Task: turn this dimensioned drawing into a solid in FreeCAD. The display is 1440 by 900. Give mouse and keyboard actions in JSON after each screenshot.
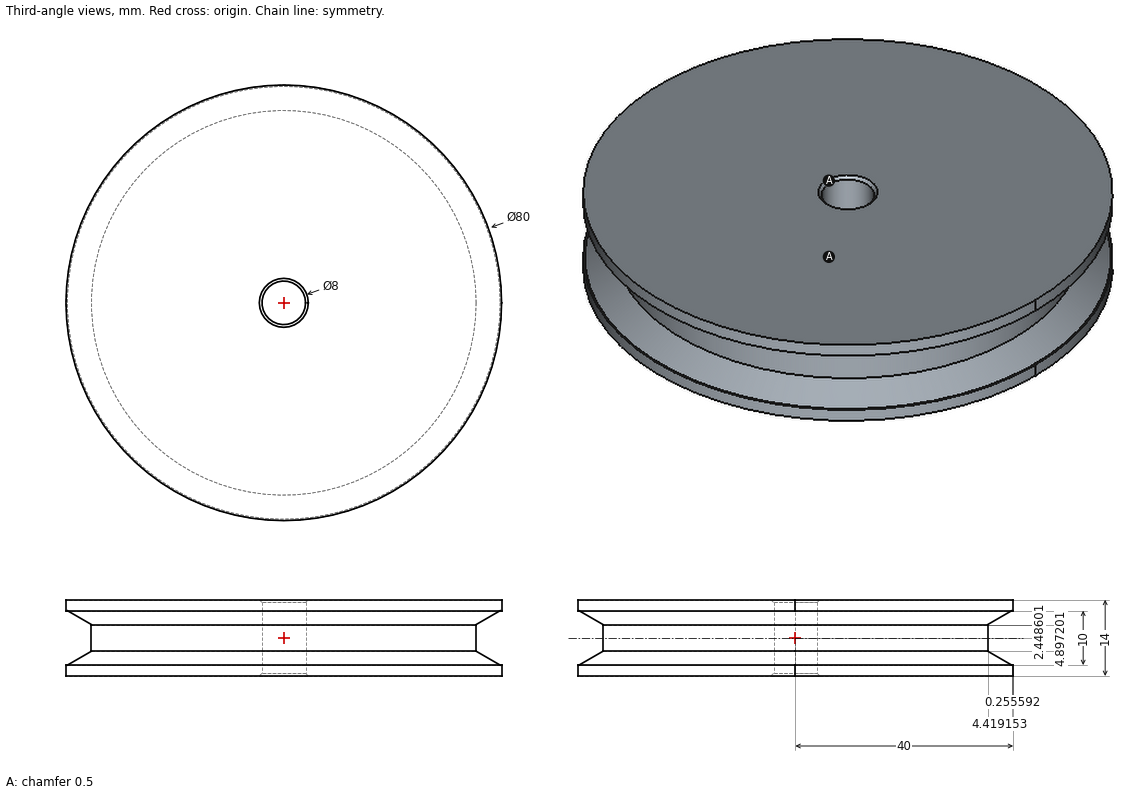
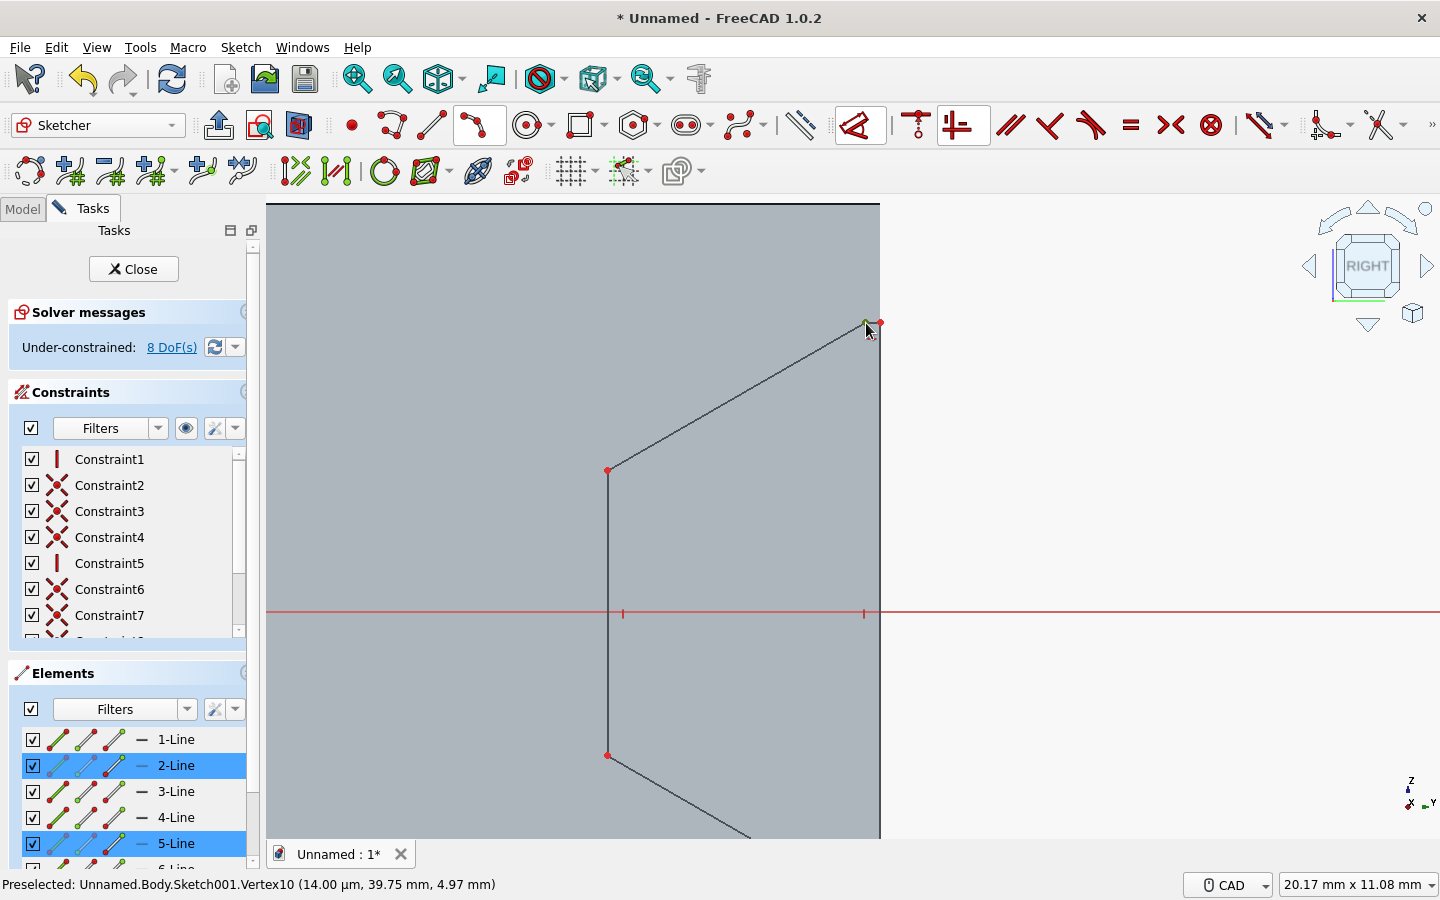
{"action": "left_click", "coordinate": [364, 612]}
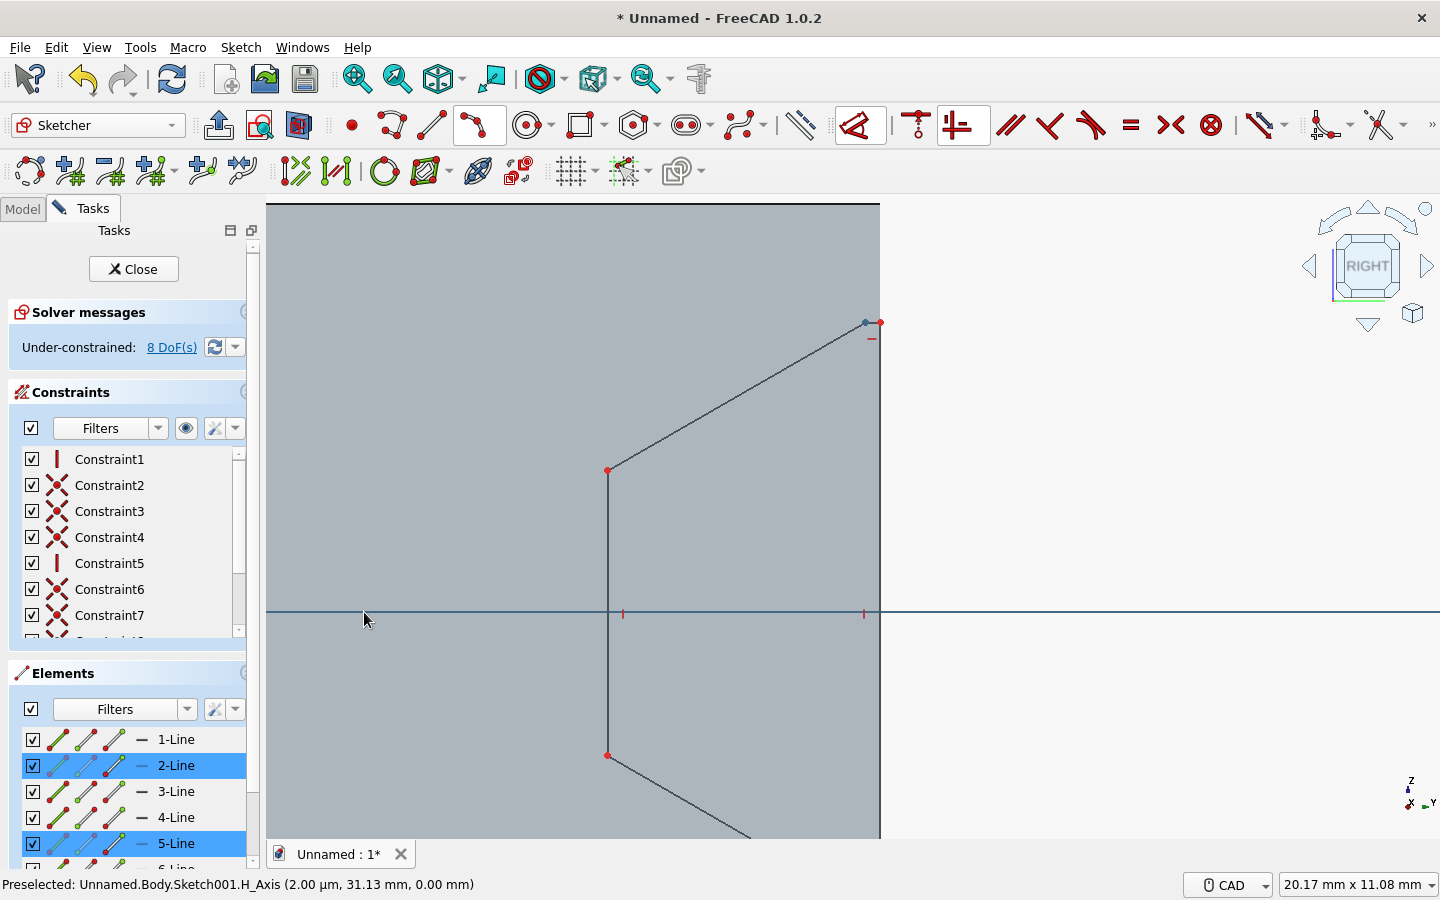
{"action": "left_click", "coordinate": [1172, 126]}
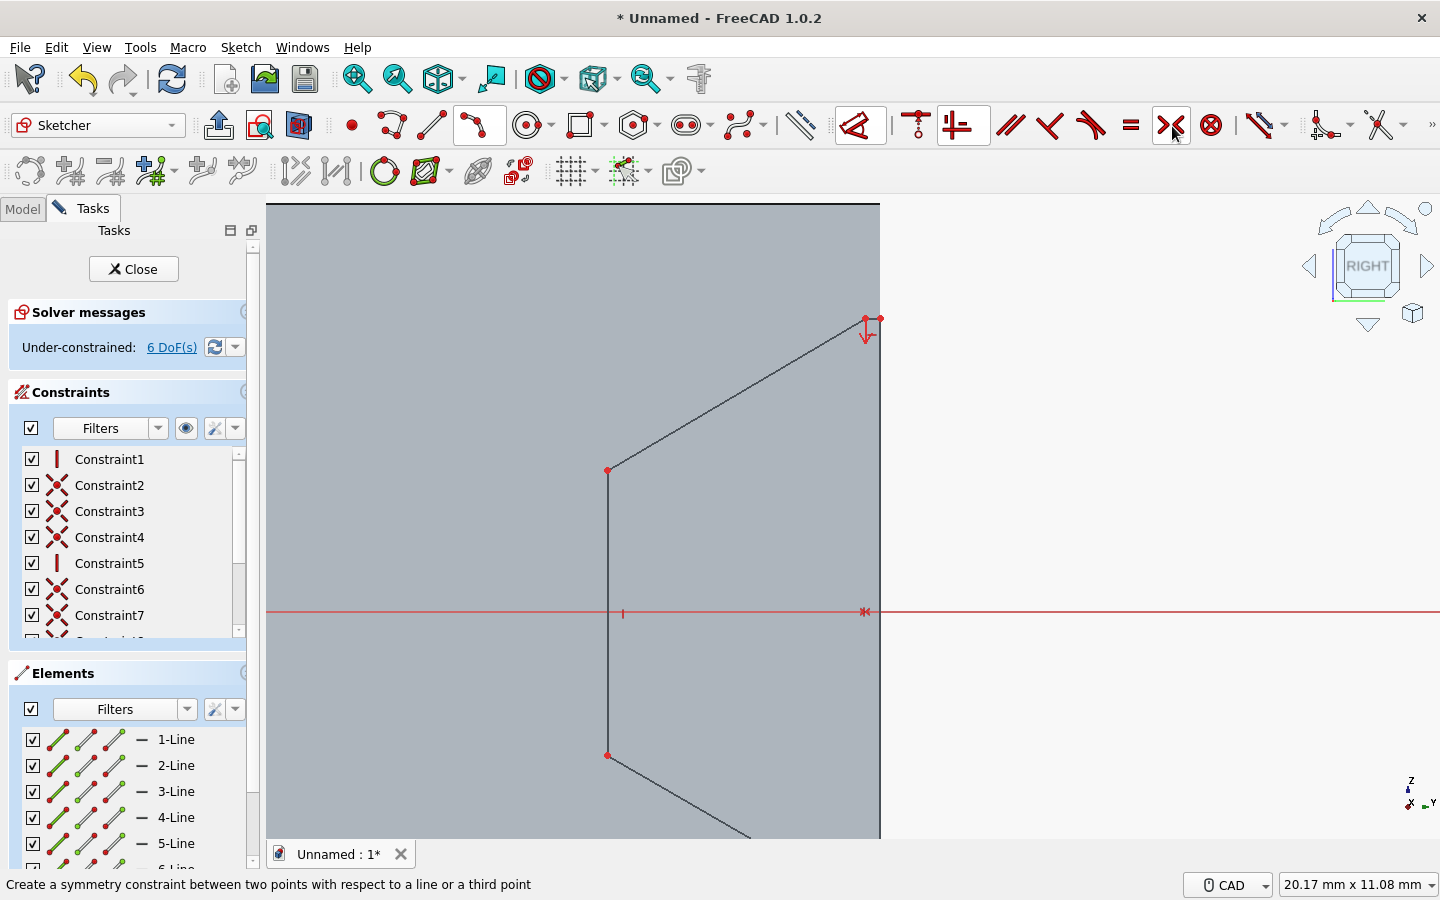
{"action": "left_click", "coordinate": [854, 126]}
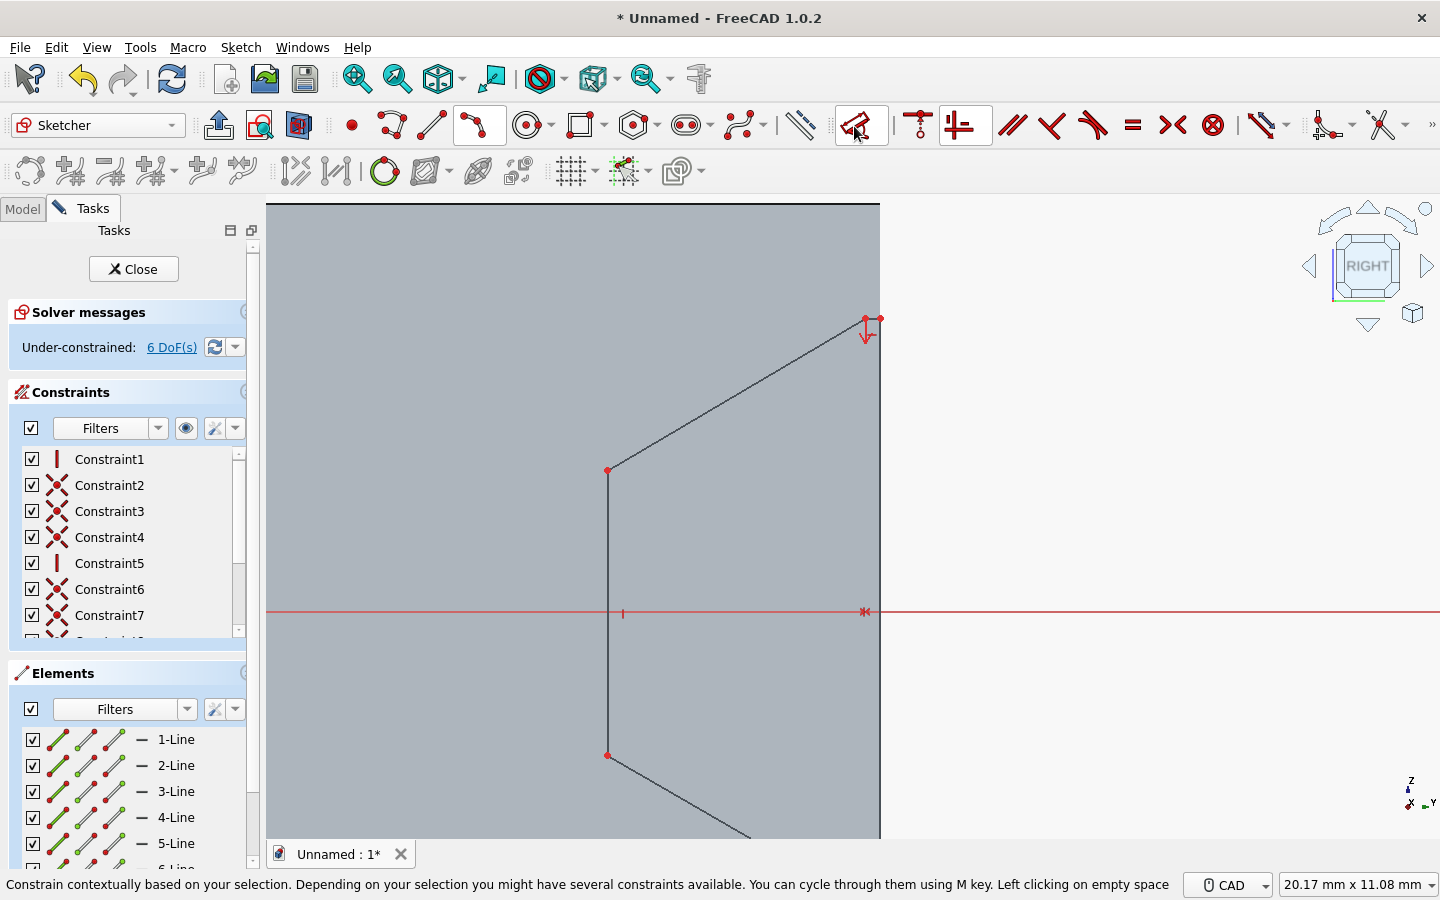
{"action": "left_click", "coordinate": [880, 729]}
{"action": "left_click", "coordinate": [914, 565]}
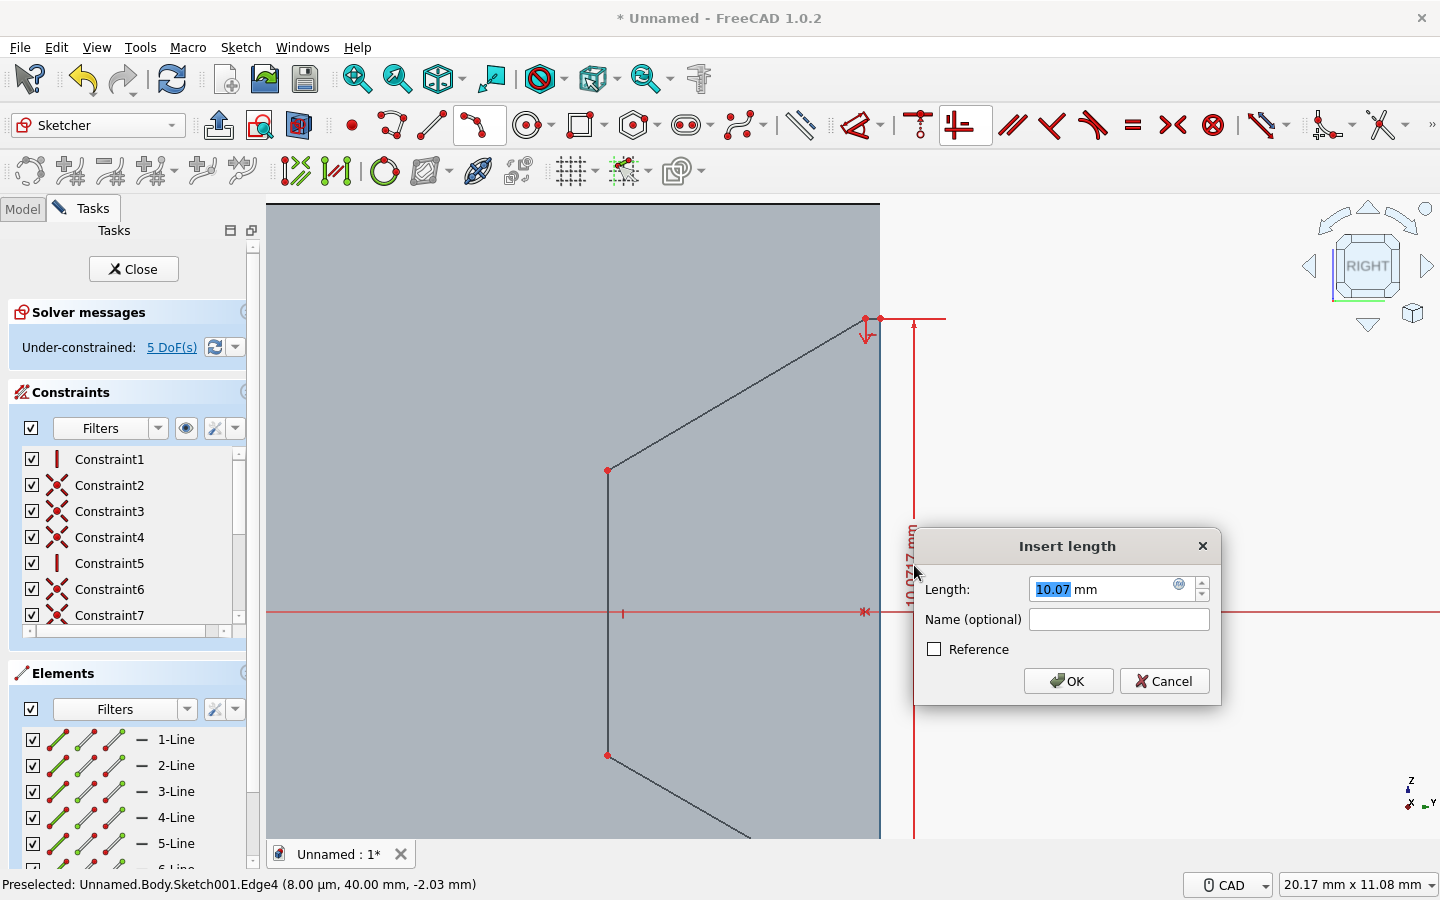
{"action": "type", "text": "10"}
{"action": "key", "text": "Return"}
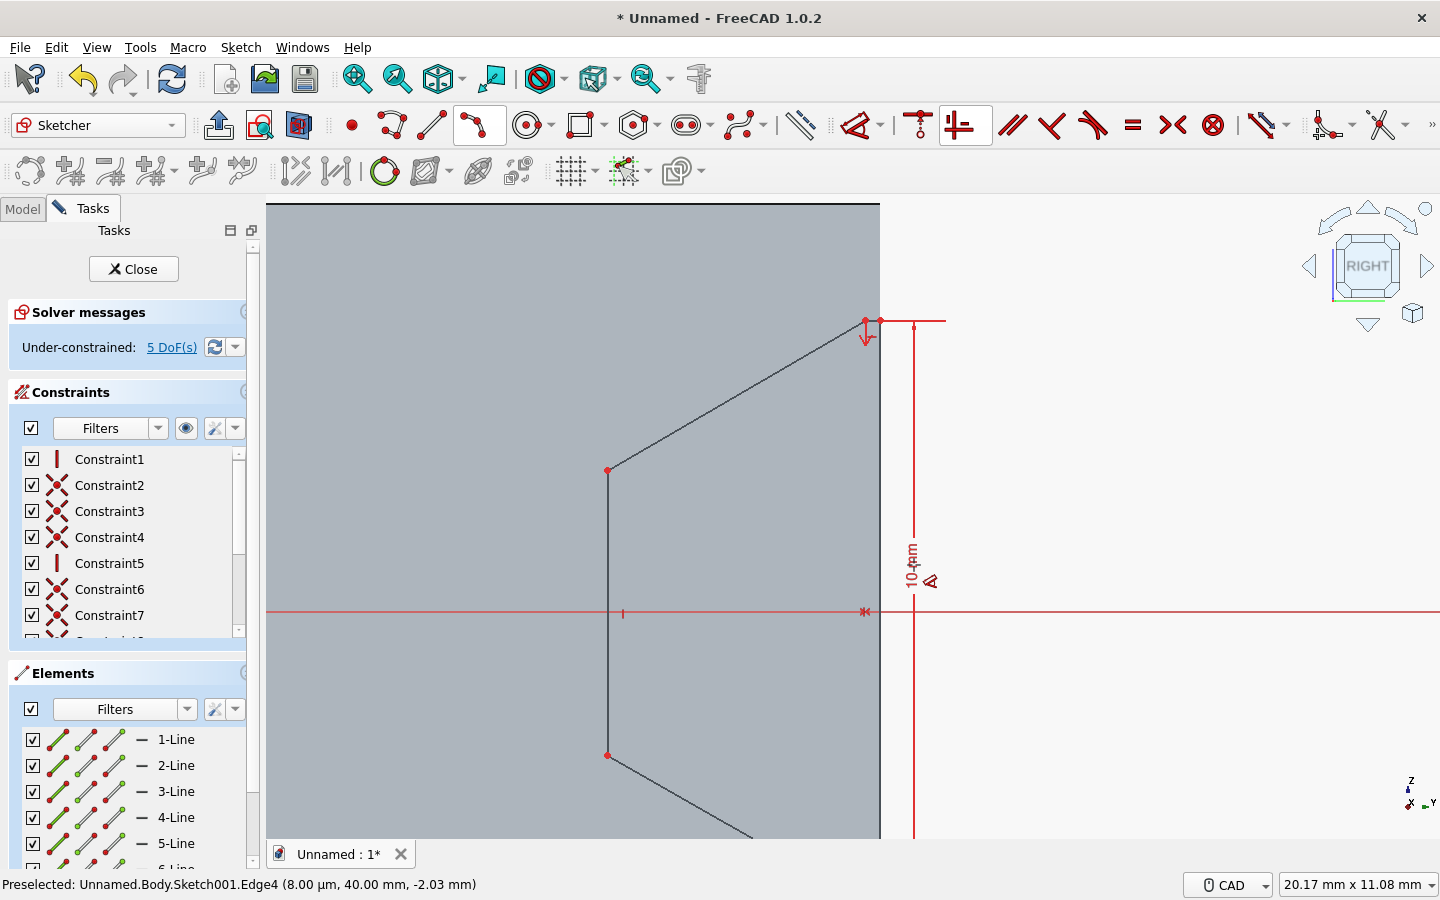
{"action": "scroll", "coordinate": [866, 323], "scroll_direction": "down", "scroll_amount": 2}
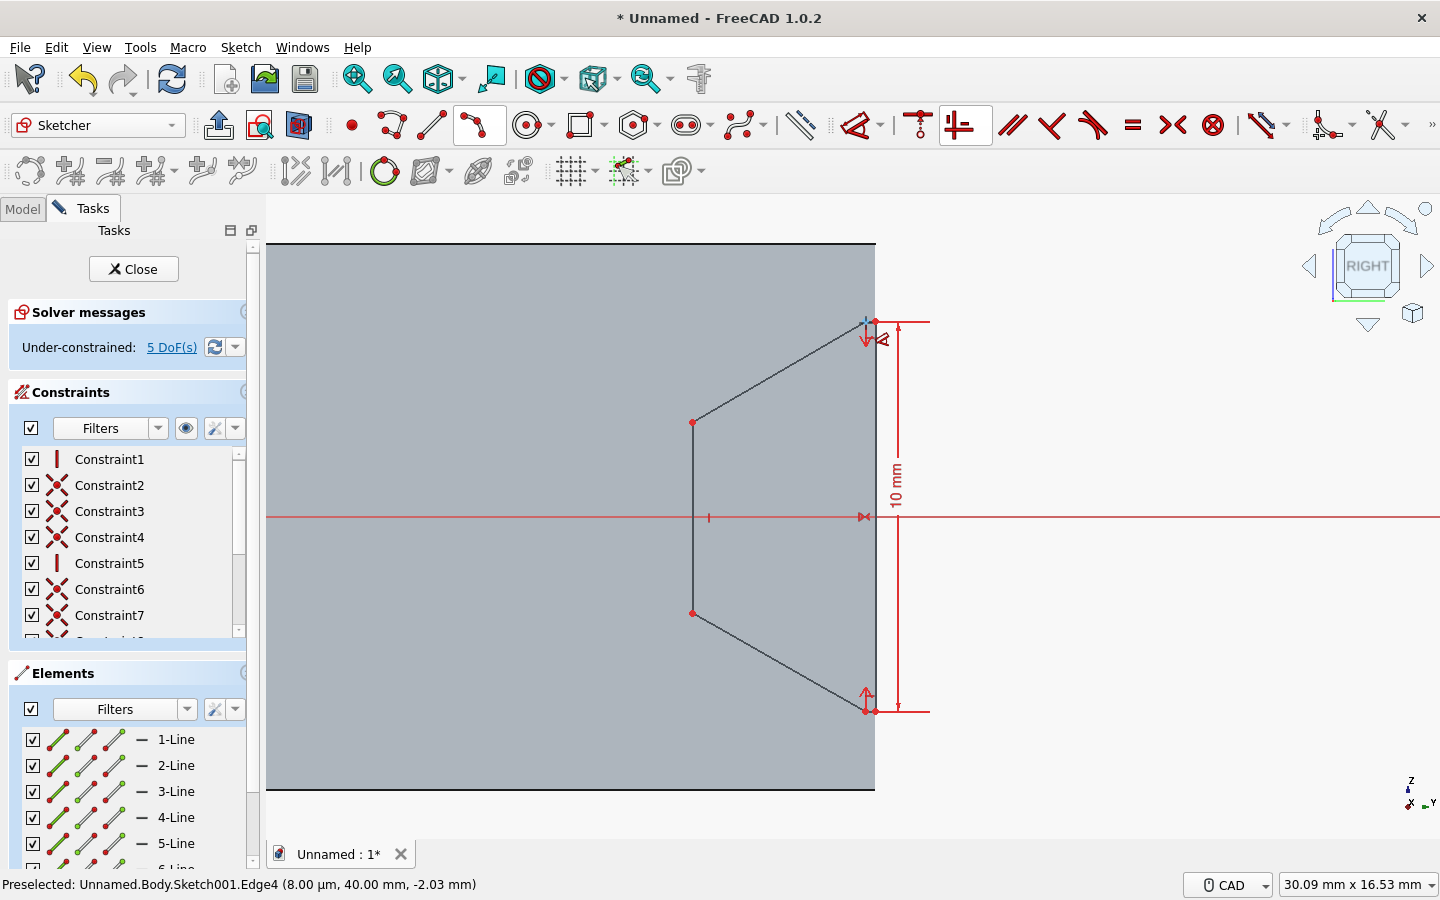
{"action": "scroll", "coordinate": [876, 712], "scroll_direction": "up", "scroll_amount": 2}